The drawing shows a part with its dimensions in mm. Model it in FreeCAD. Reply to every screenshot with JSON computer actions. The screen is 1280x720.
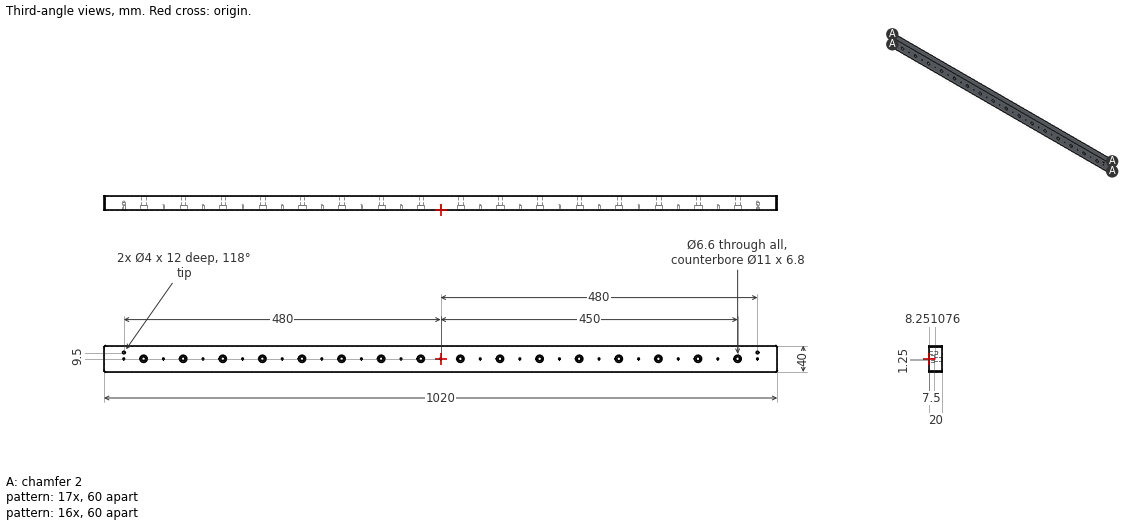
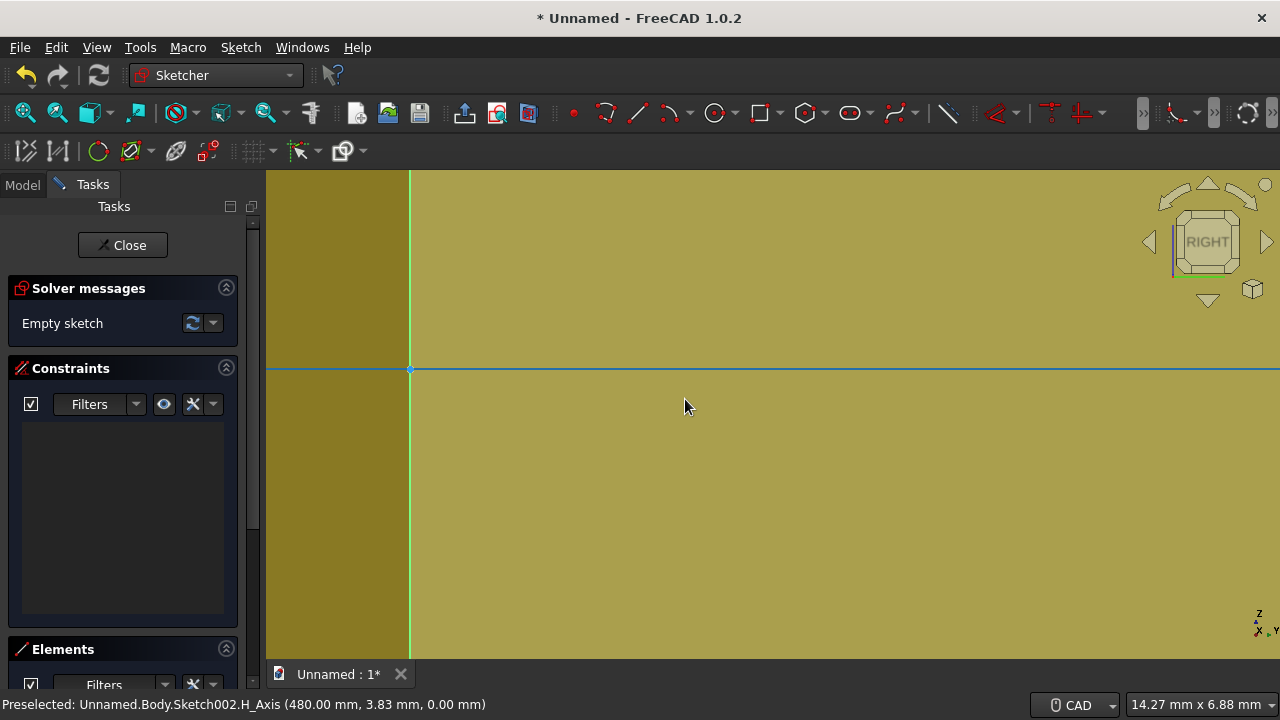
{"action": "left_click", "coordinate": [606, 114]}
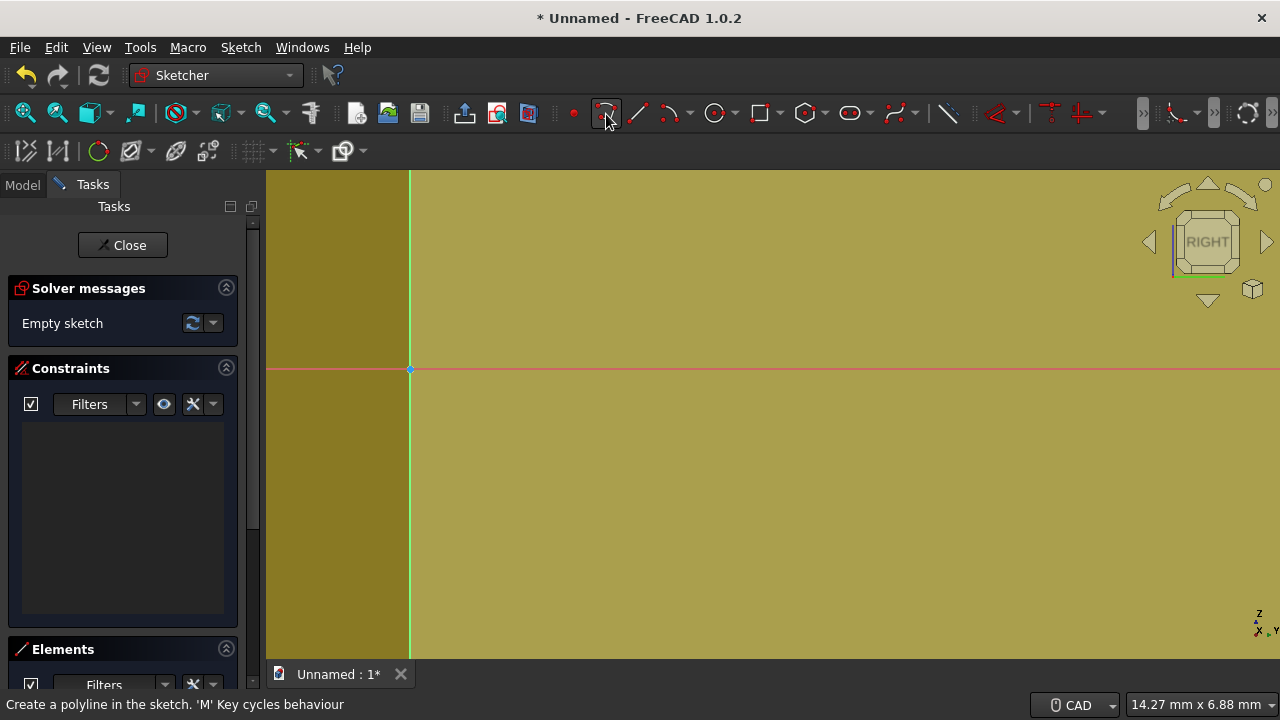
{"action": "left_click", "coordinate": [410, 369]}
{"action": "left_click", "coordinate": [419, 458]}
{"action": "left_click", "coordinate": [943, 458]}
{"action": "left_click", "coordinate": [997, 378]}
{"action": "left_click", "coordinate": [410, 369]}
{"action": "key", "text": "Escape"}
{"action": "key", "text": "Escape"}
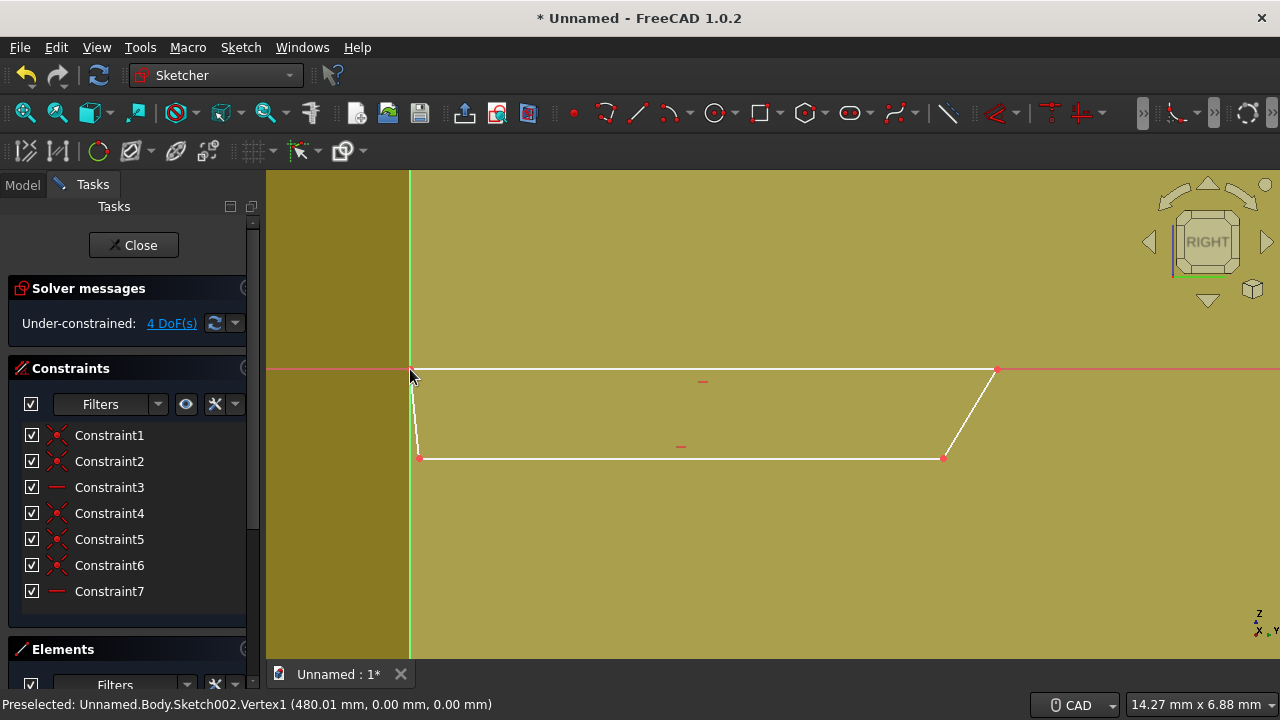
{"action": "left_click", "coordinate": [413, 396]}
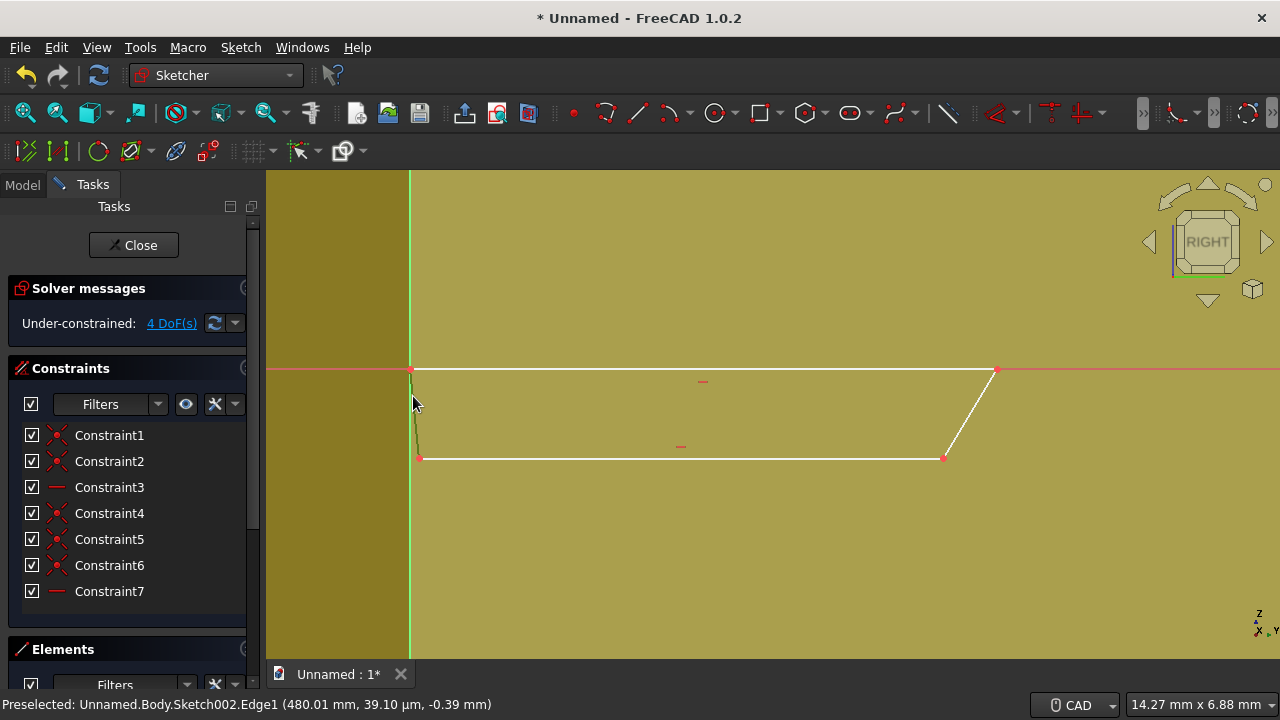
{"action": "key", "text": "v"}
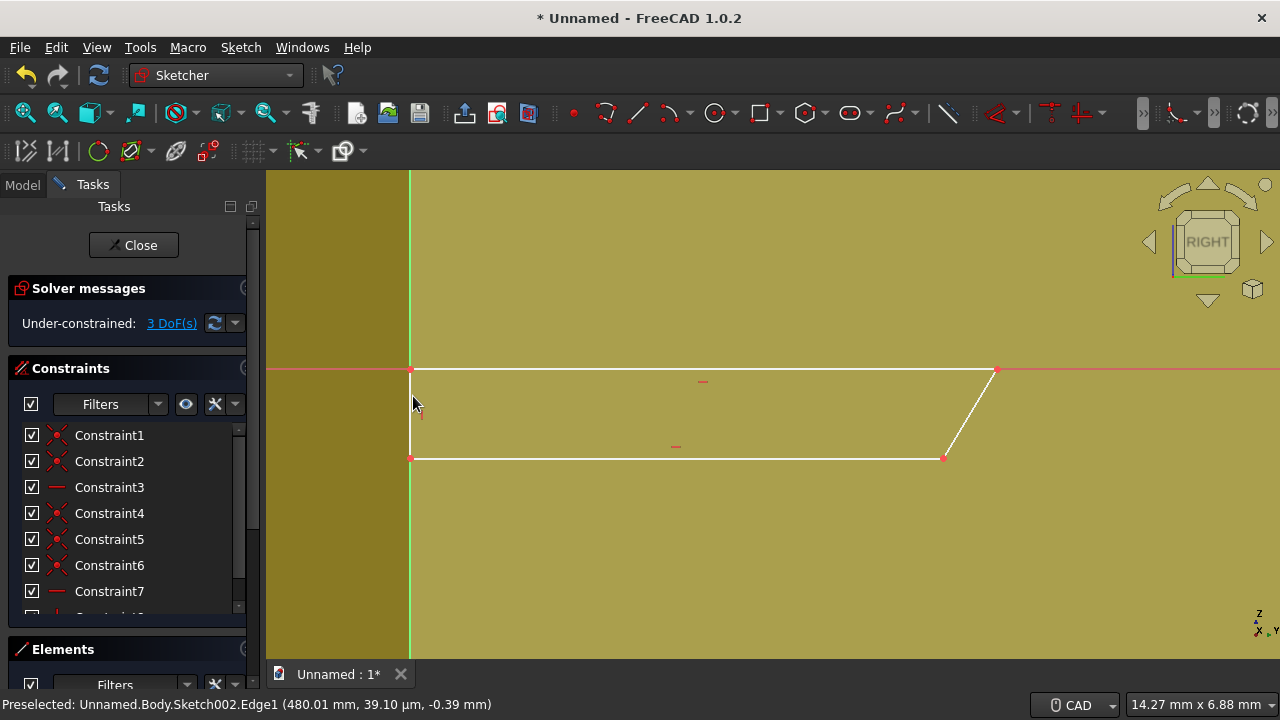
{"action": "key", "text": "d"}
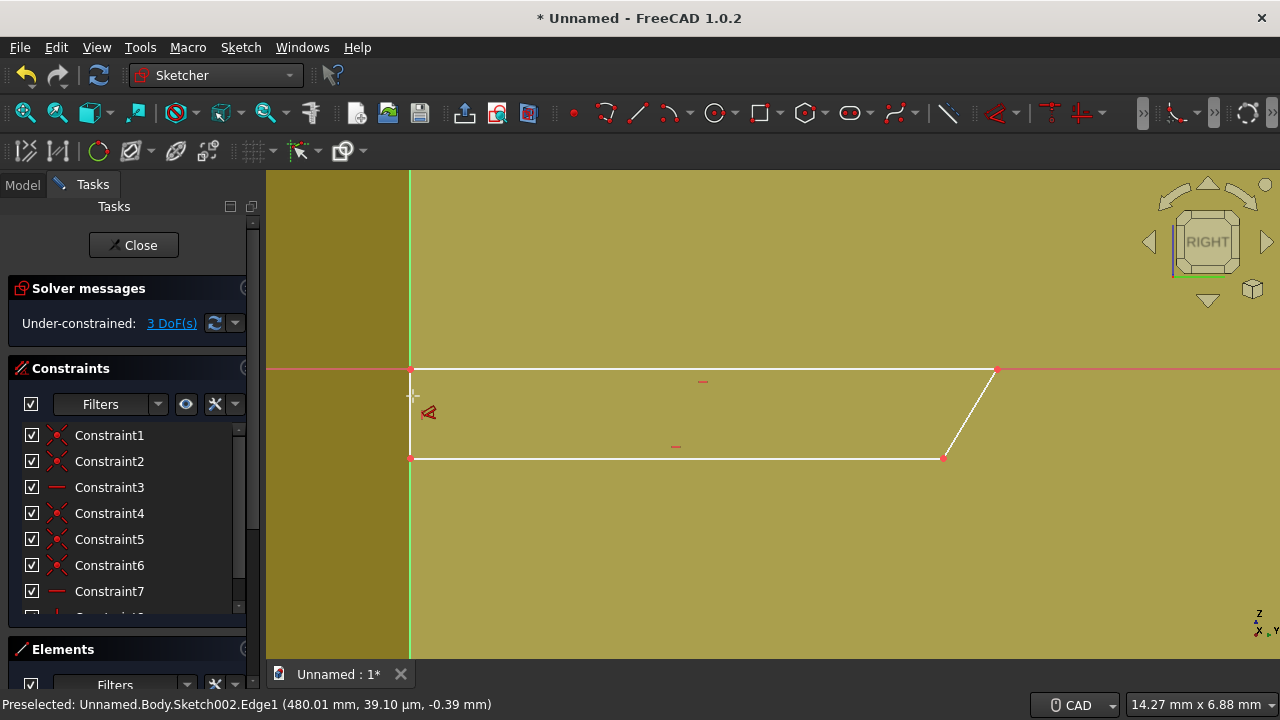
{"action": "left_click", "coordinate": [570, 459]}
{"action": "left_click", "coordinate": [677, 493]}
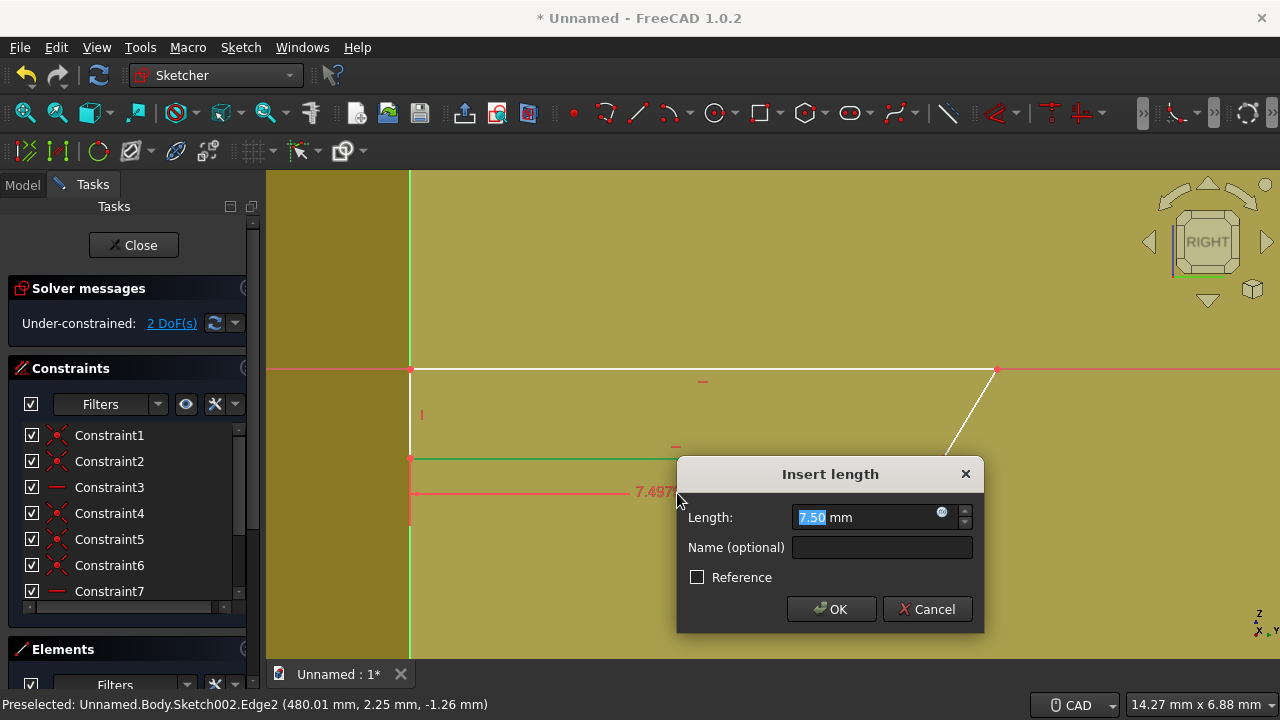
{"action": "type", "text": "7.5"}
{"action": "key", "text": "Return"}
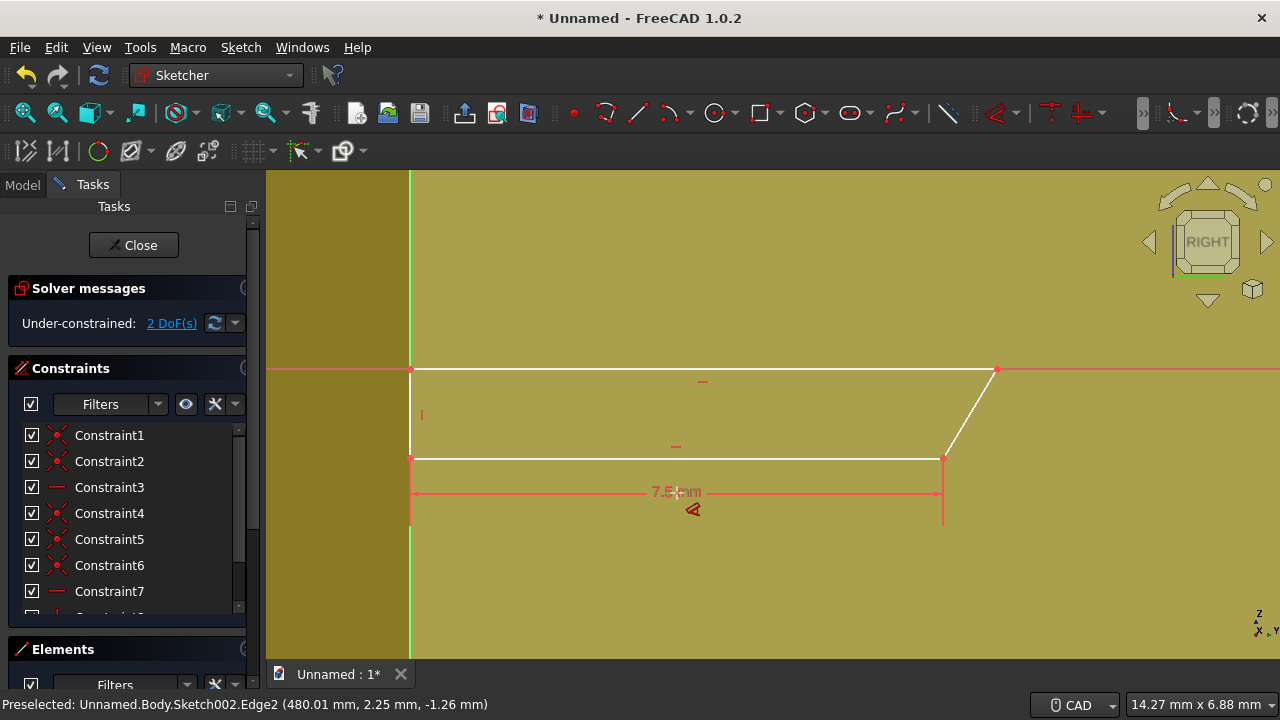
{"action": "left_click", "coordinate": [410, 396]}
{"action": "left_click", "coordinate": [376, 414]}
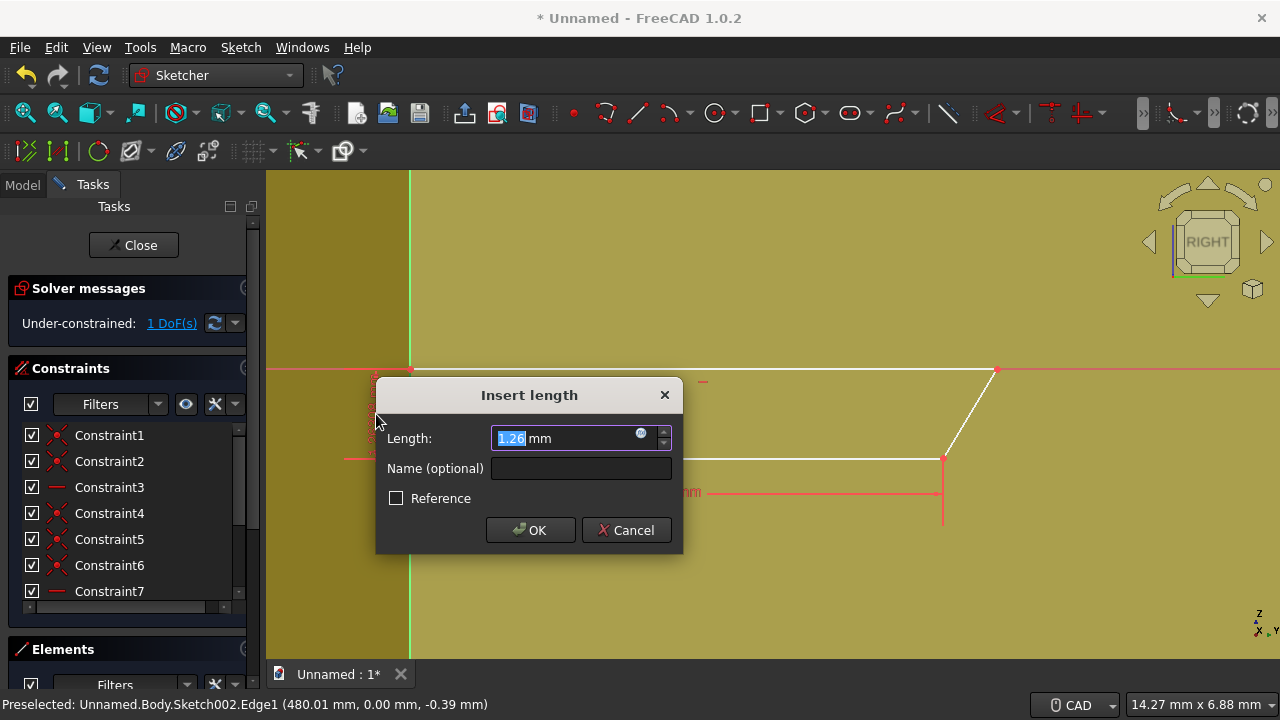
{"action": "type", "text": "1.25"}
{"action": "key", "text": "Return"}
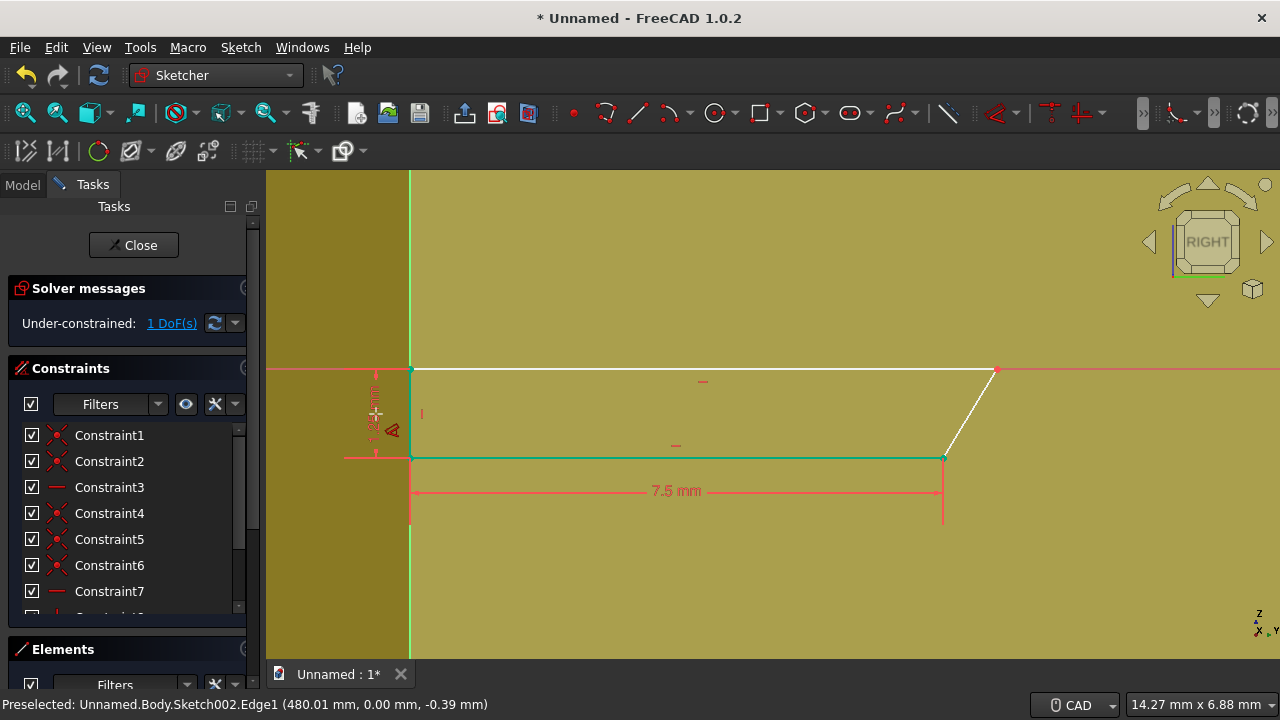
{"action": "left_click", "coordinate": [821, 369]}
{"action": "left_click", "coordinate": [704, 335]}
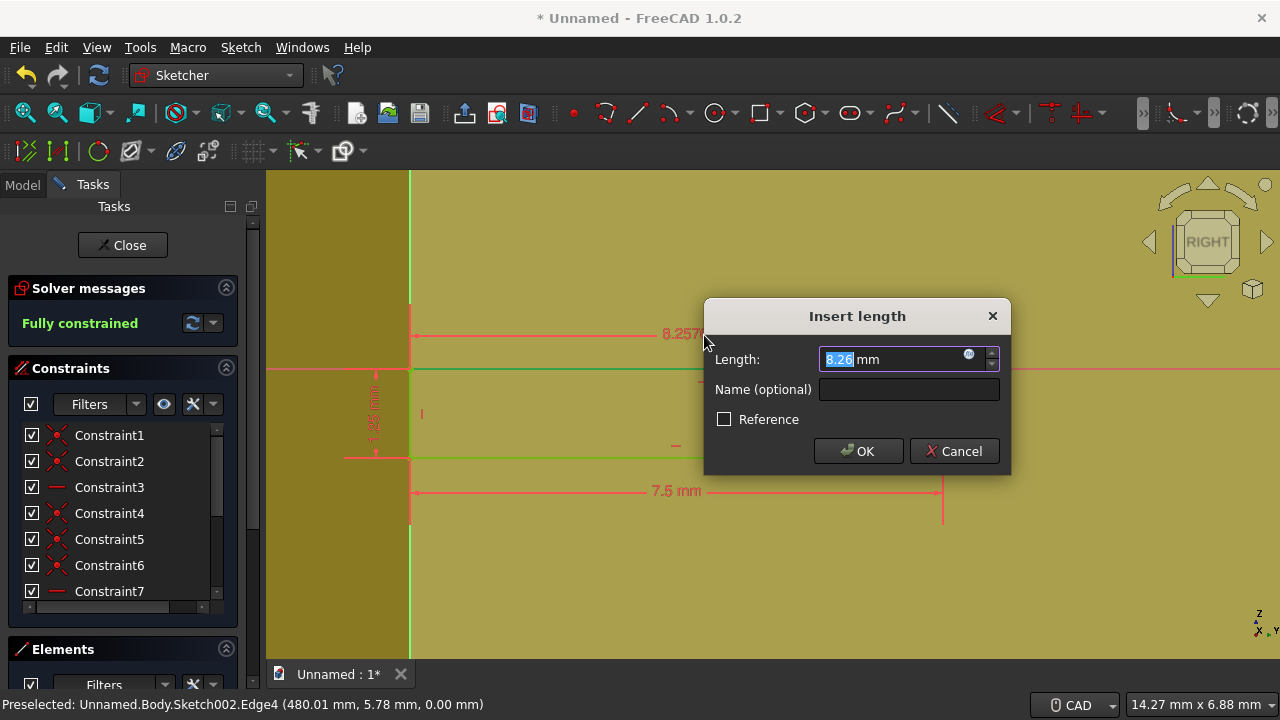
{"action": "type", "text": "8.251076"}
{"action": "key", "text": "Return"}
{"action": "key", "text": "Escape"}